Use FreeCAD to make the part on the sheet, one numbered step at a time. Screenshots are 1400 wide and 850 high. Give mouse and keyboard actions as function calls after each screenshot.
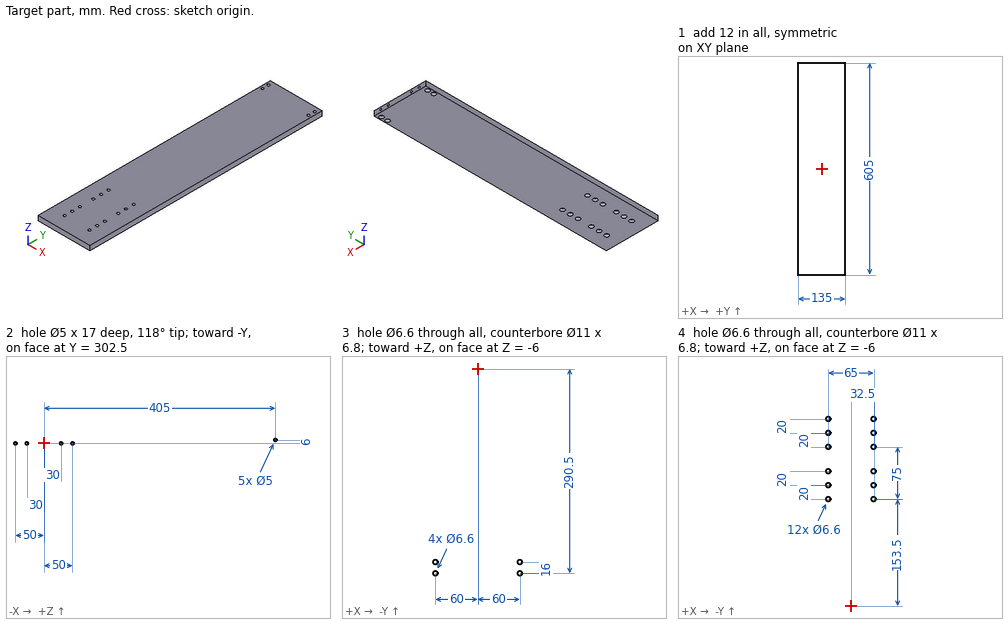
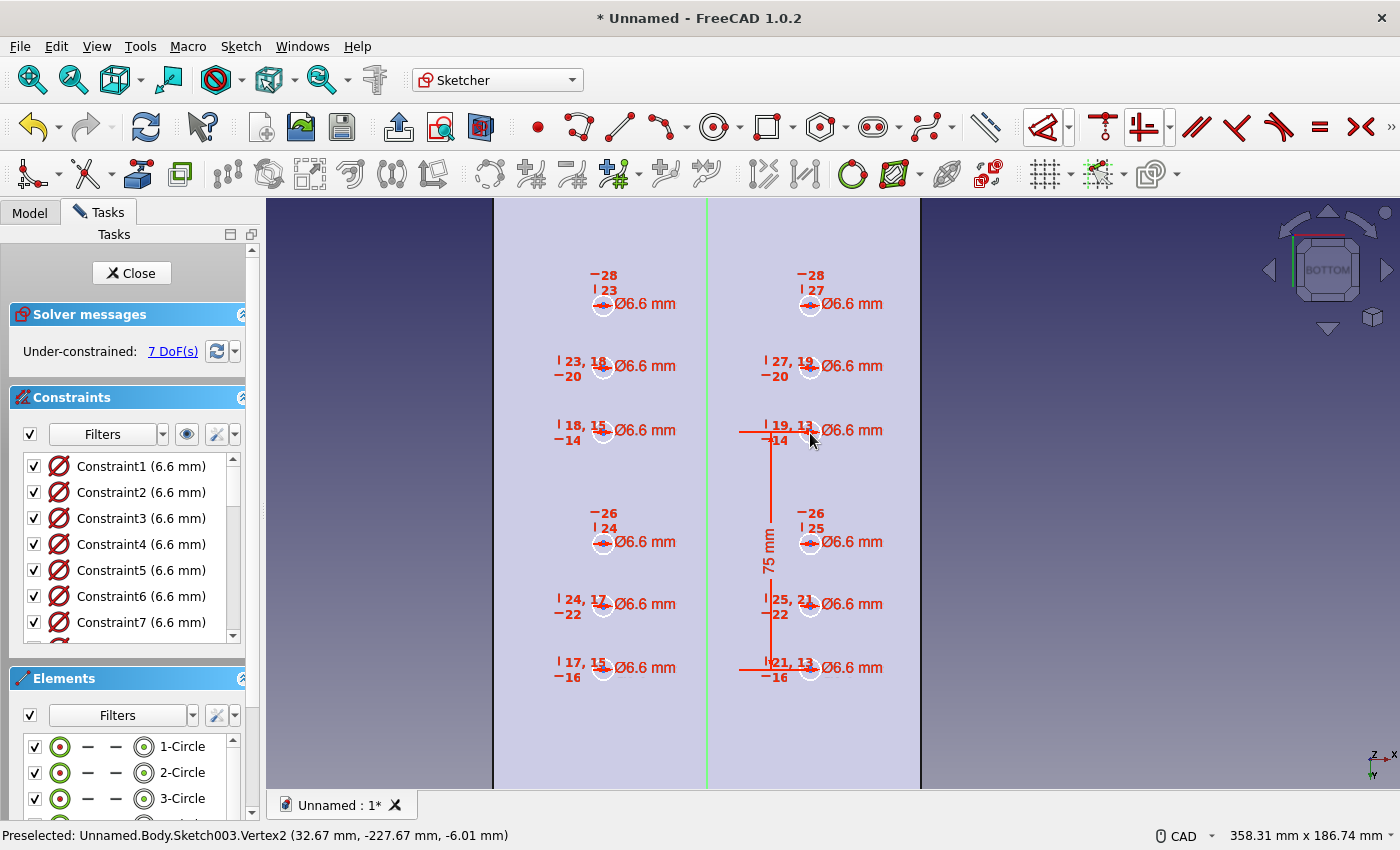
click(810, 432)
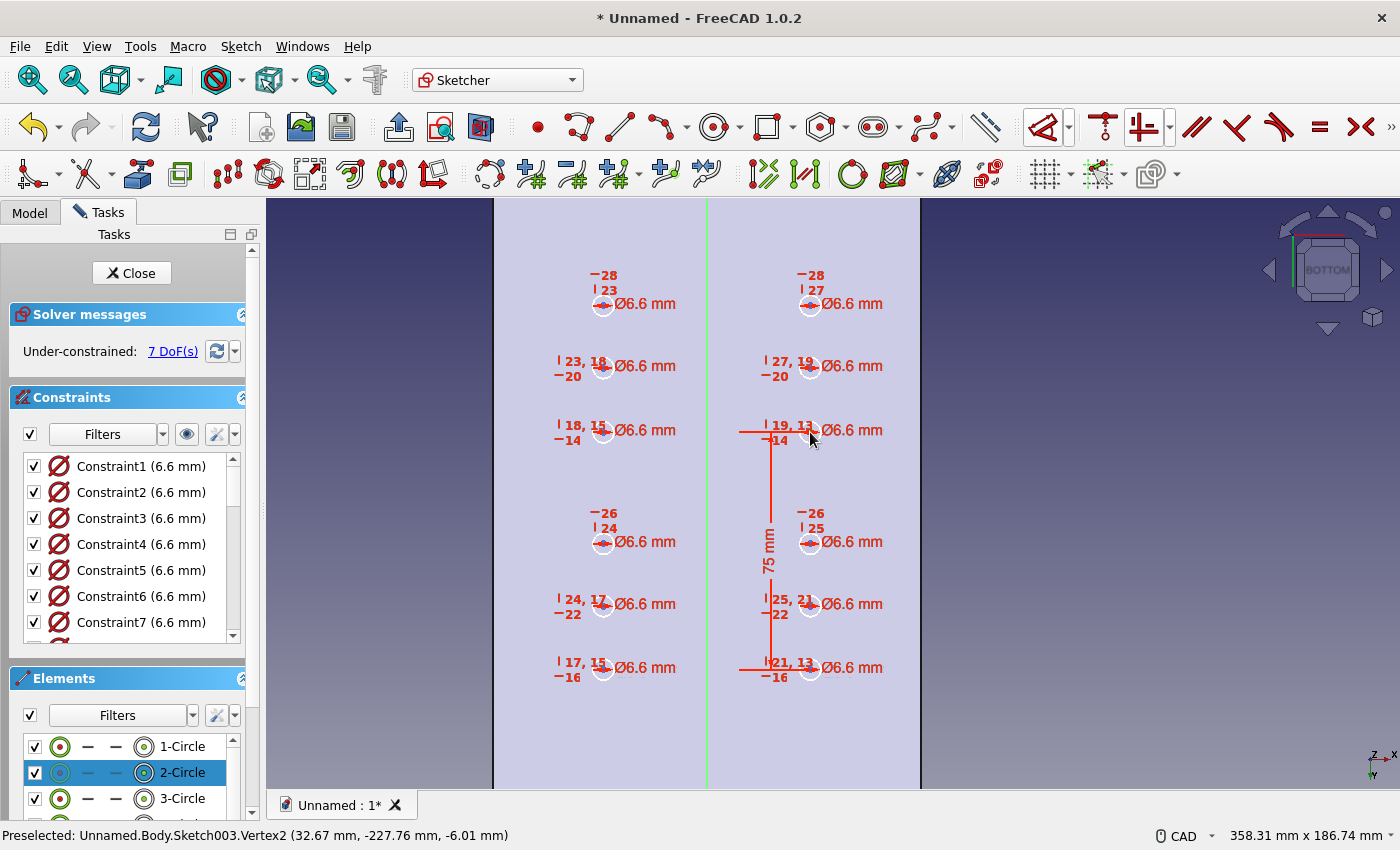
click(603, 432)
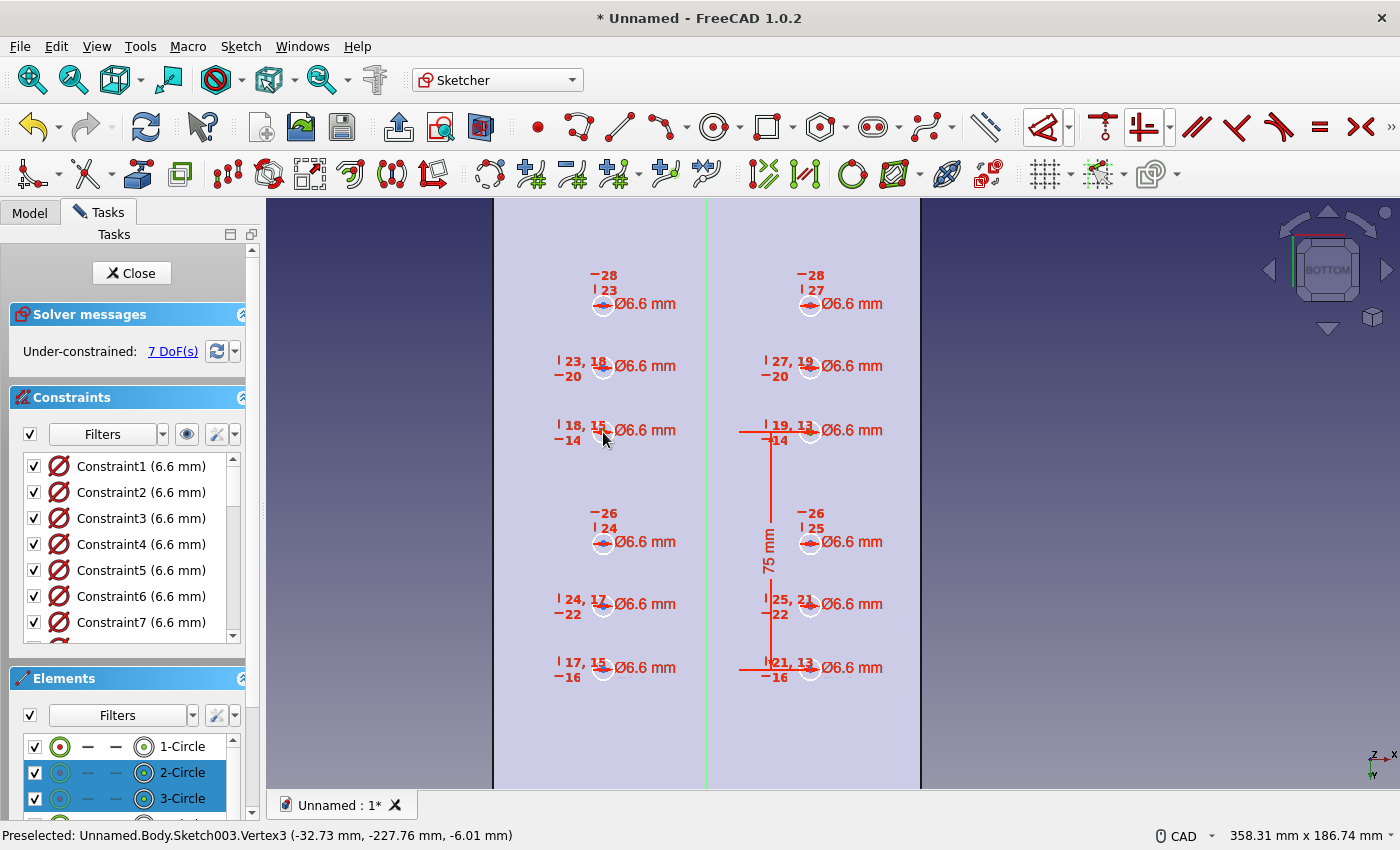
click(1068, 128)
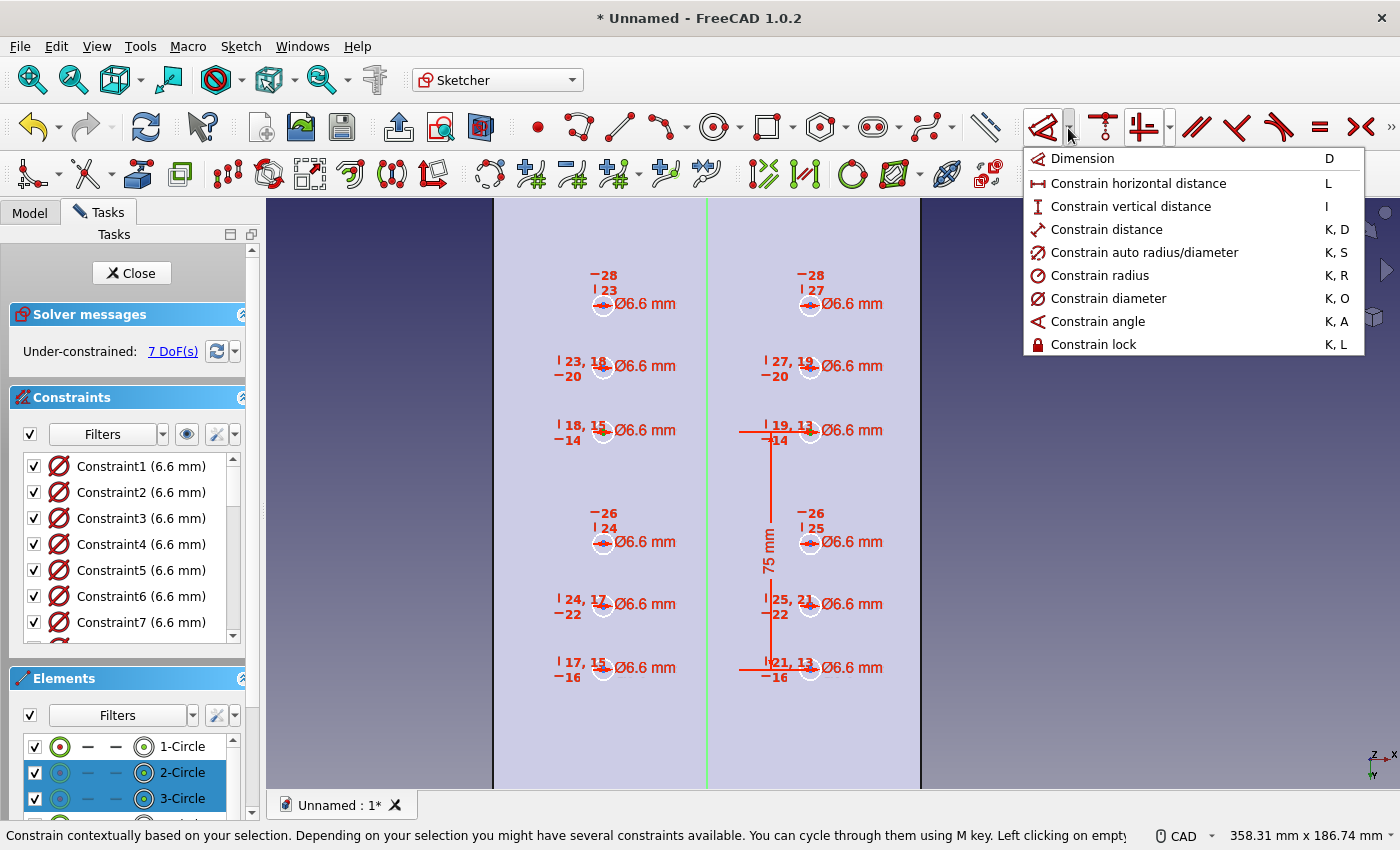
click(1194, 184)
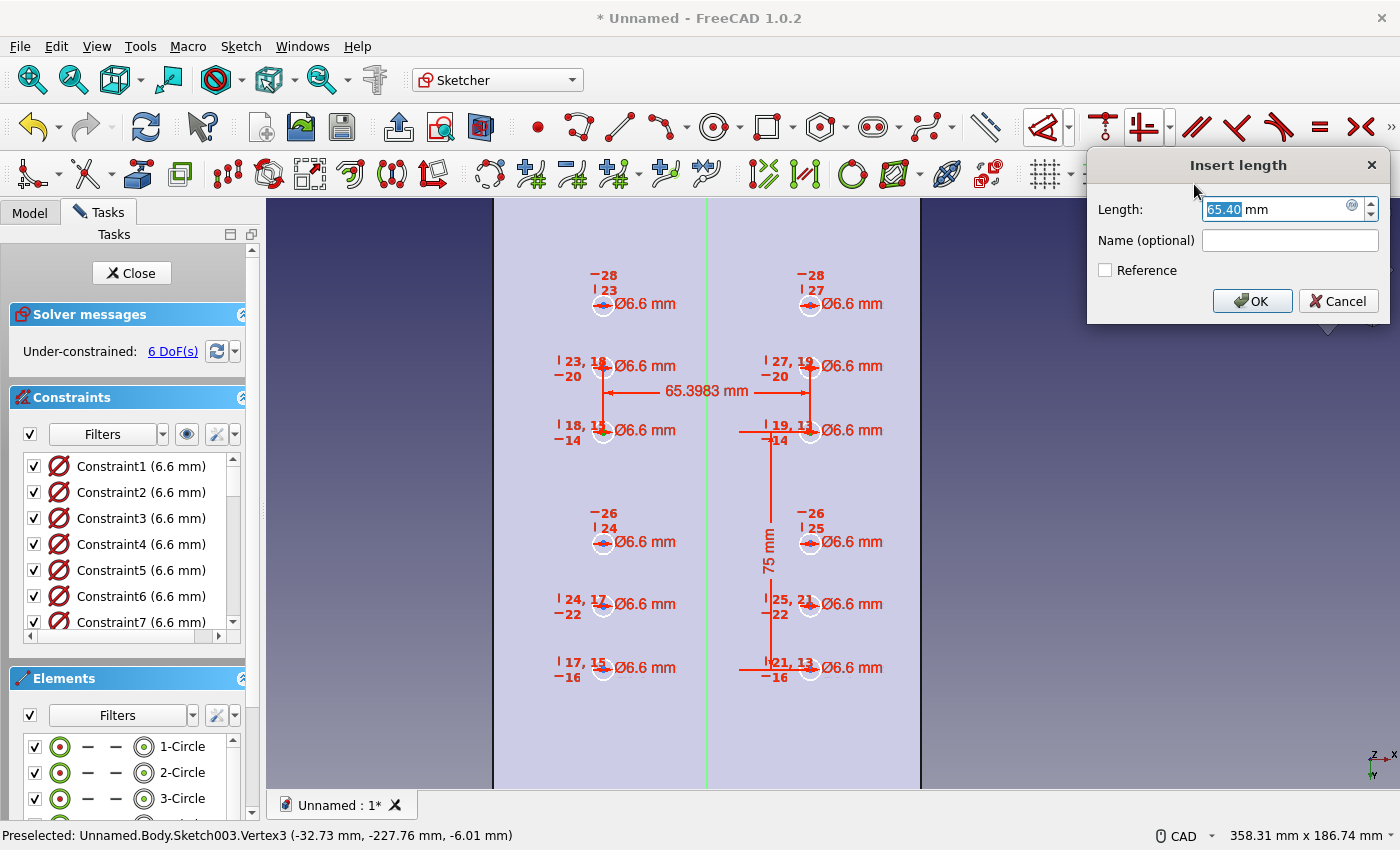
text(65)
key(Return)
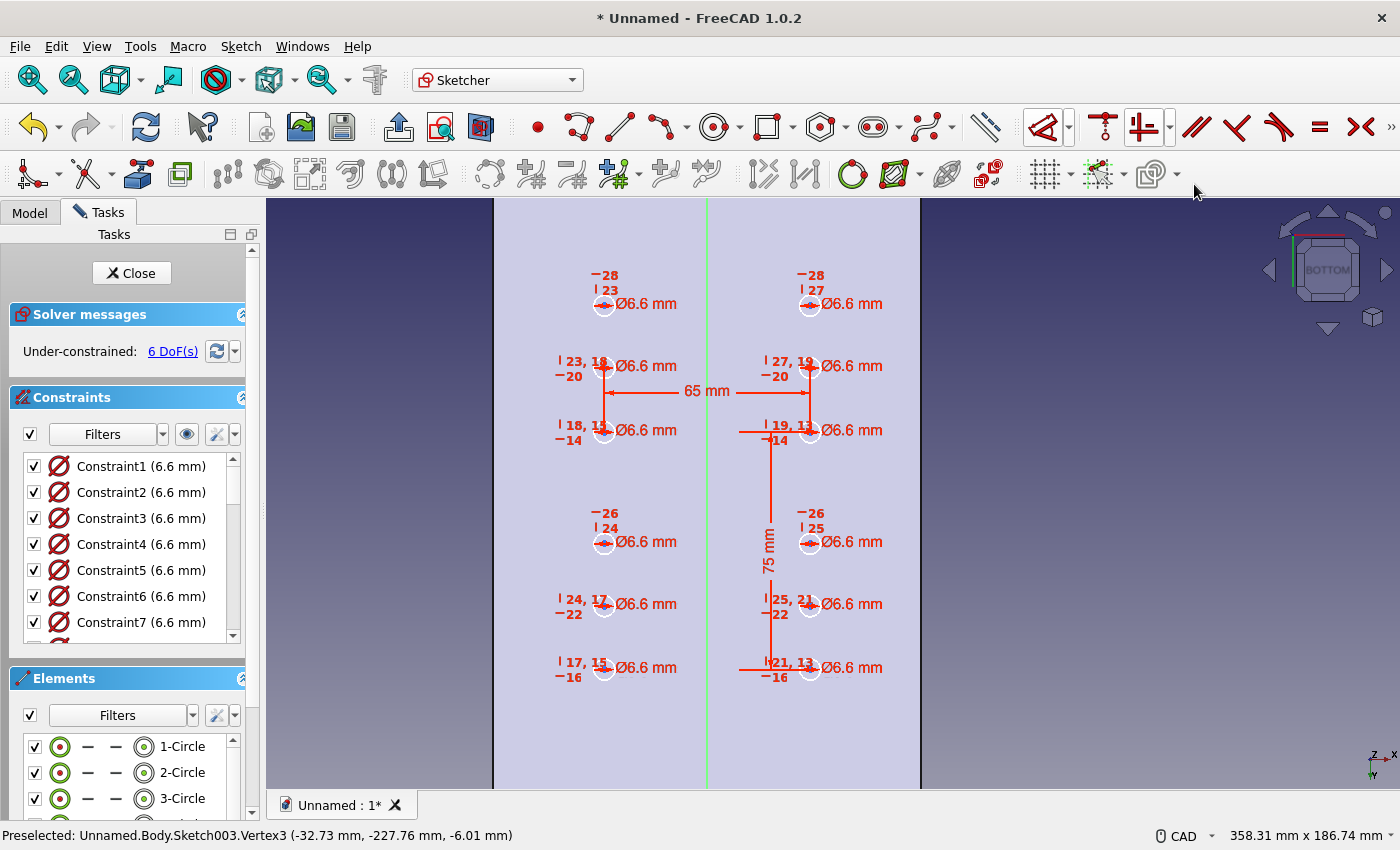
click(604, 670)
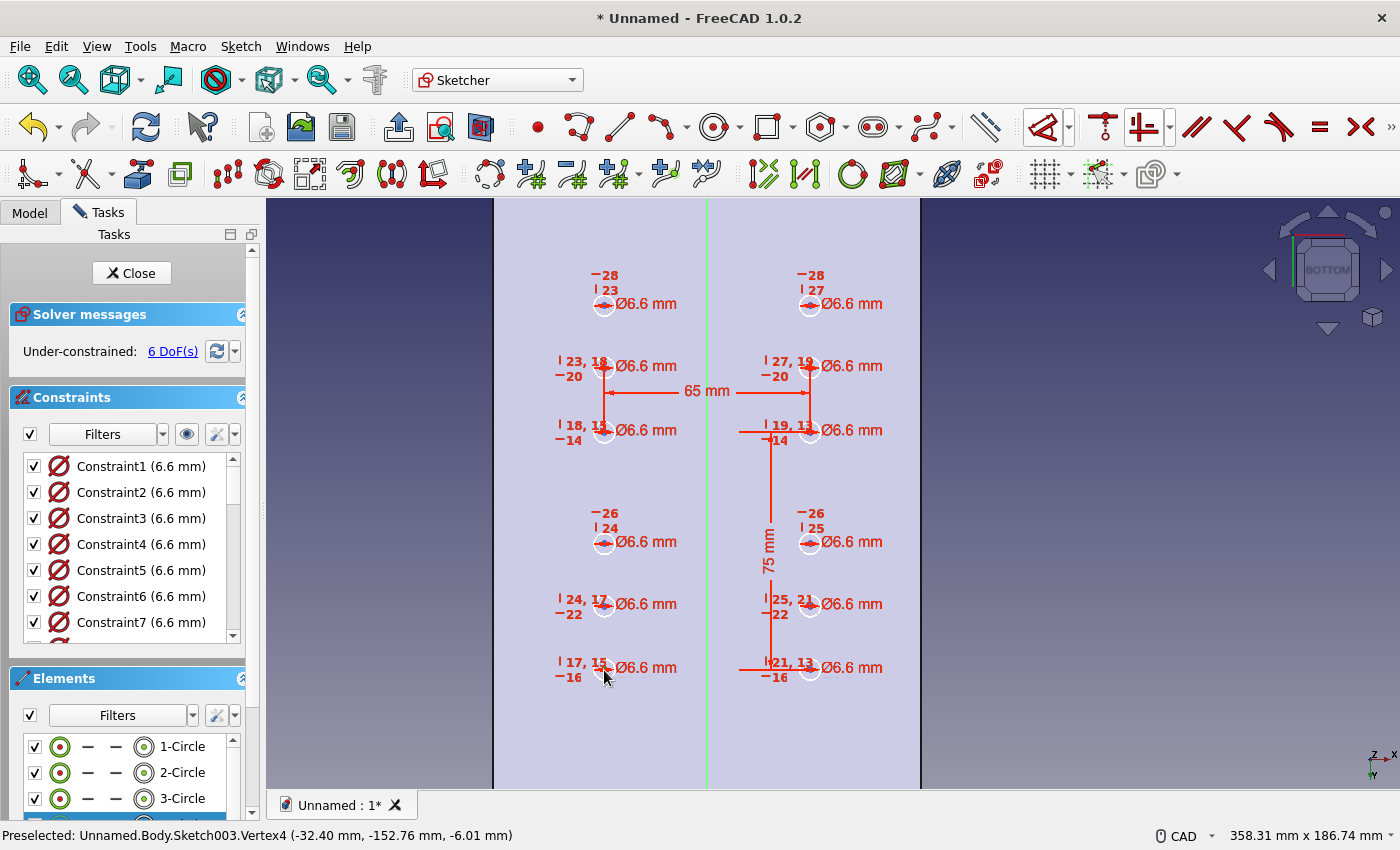
click(604, 606)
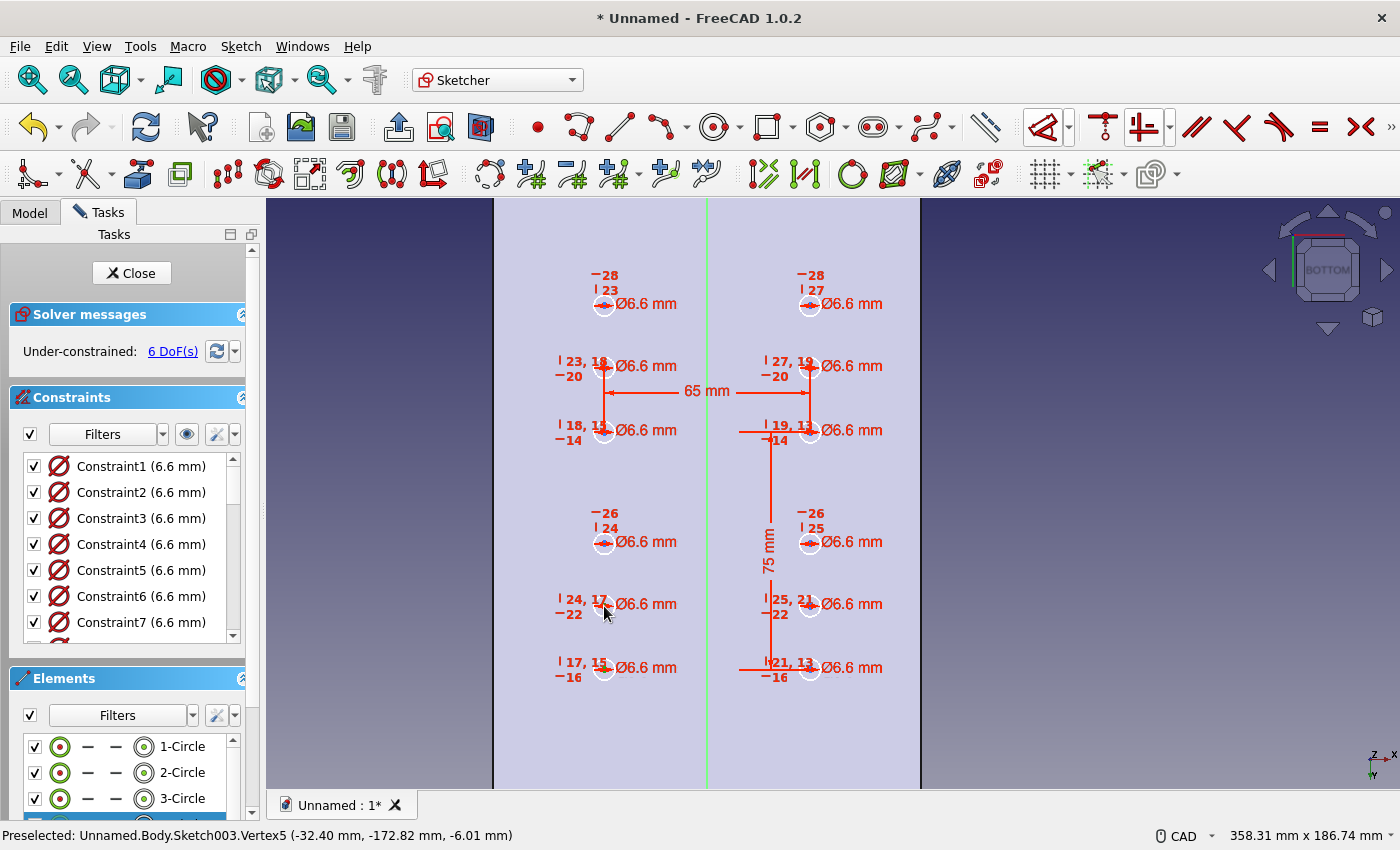
key(i)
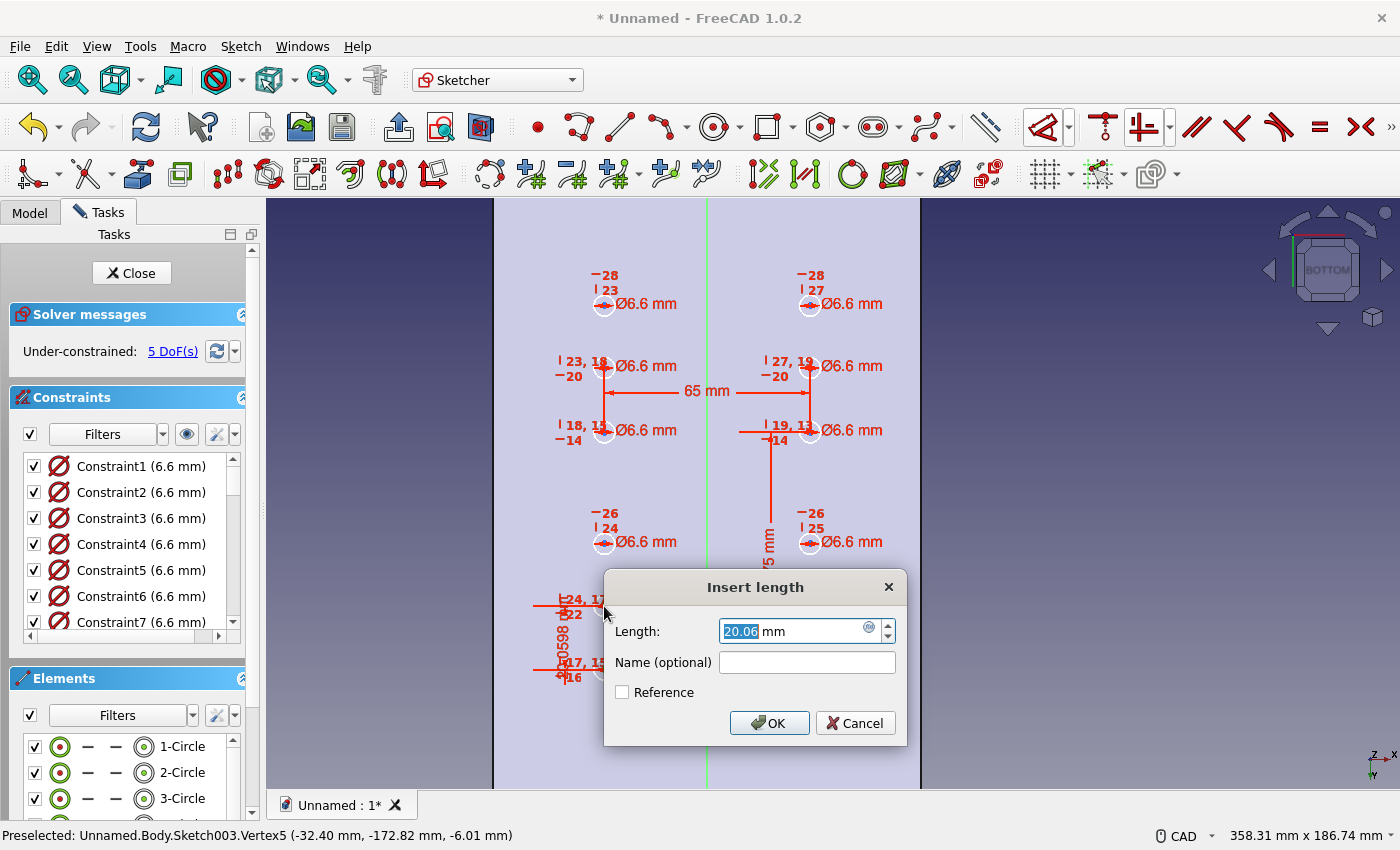
text(20)
key(Return)